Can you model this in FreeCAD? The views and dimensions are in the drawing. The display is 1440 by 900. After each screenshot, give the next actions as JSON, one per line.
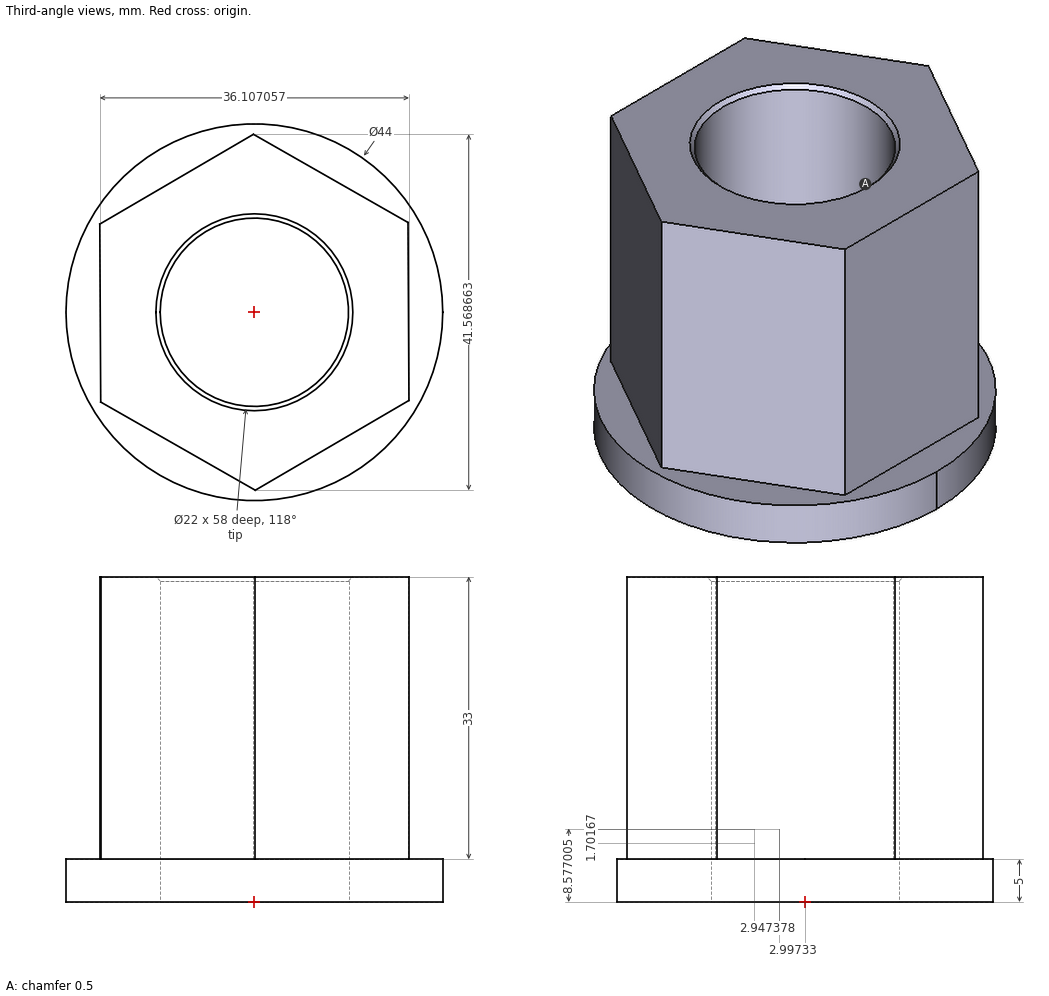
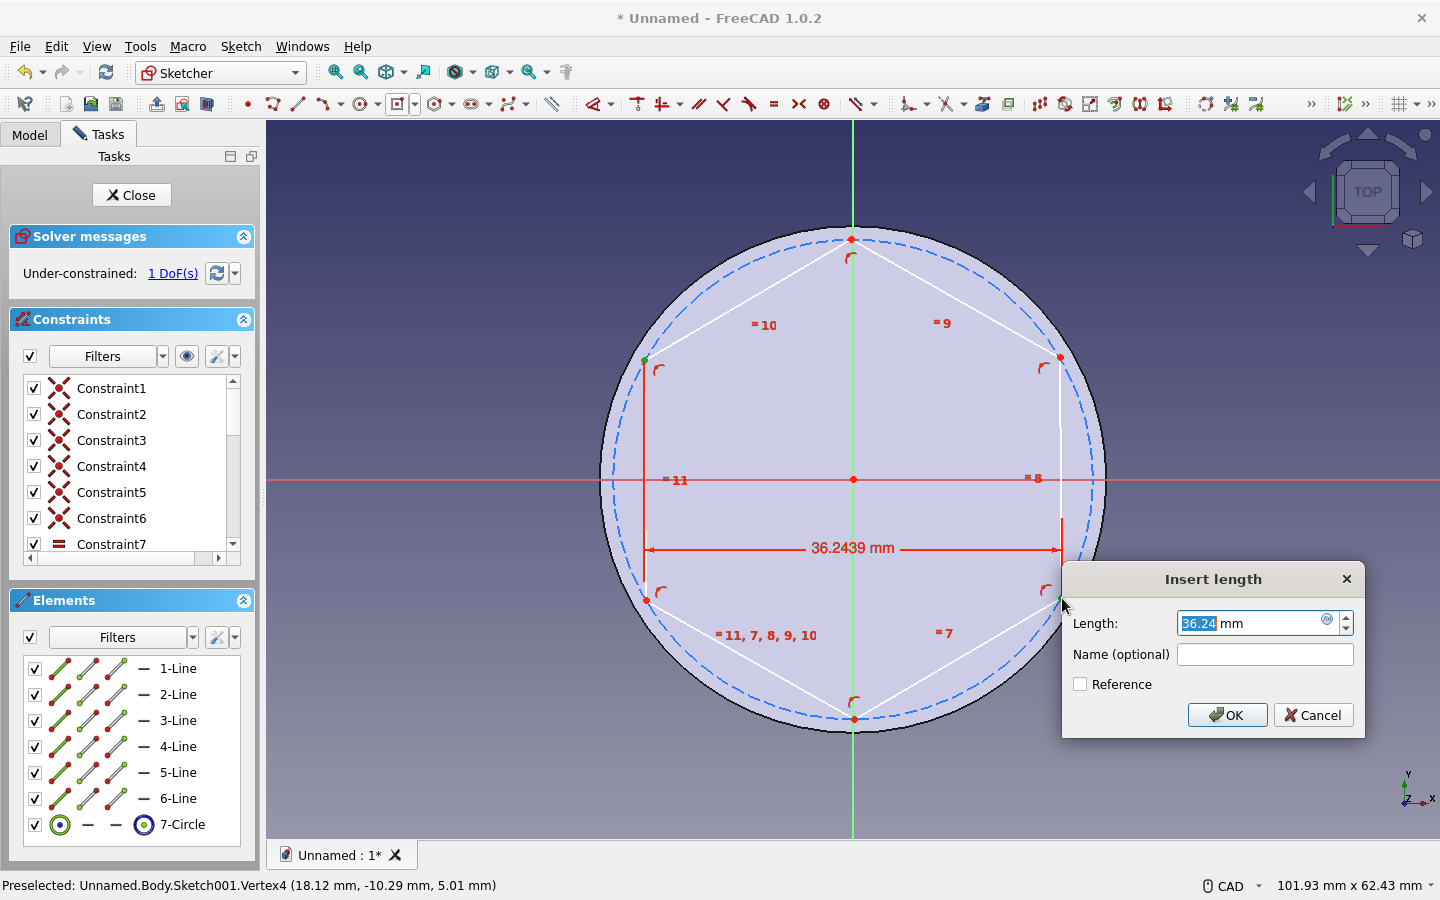
{"action": "type", "text": "36.107057"}
{"action": "key", "text": "Return"}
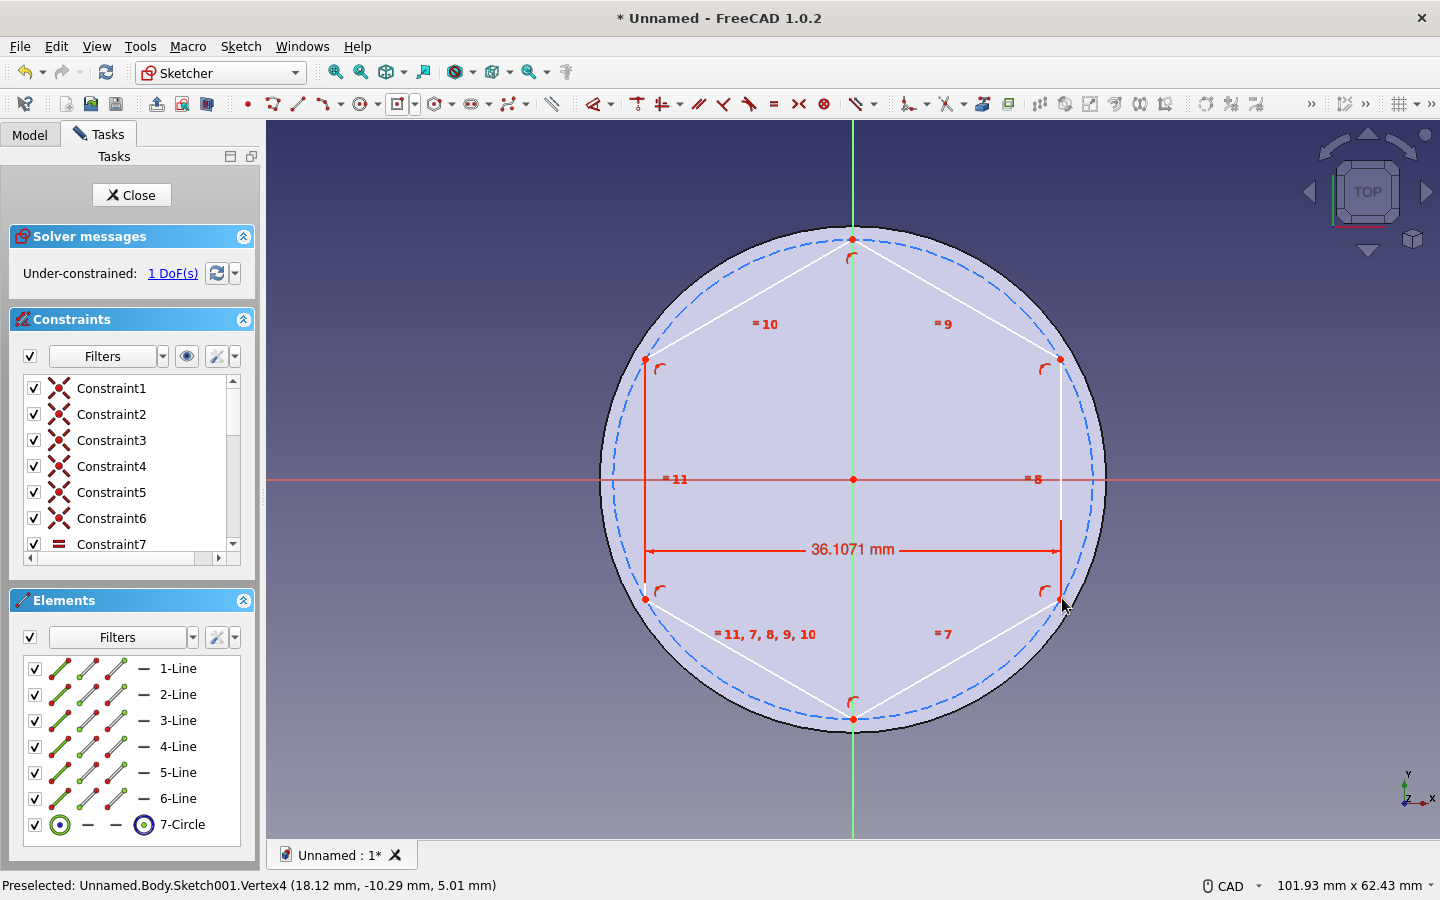
{"action": "left_click", "coordinate": [853, 720]}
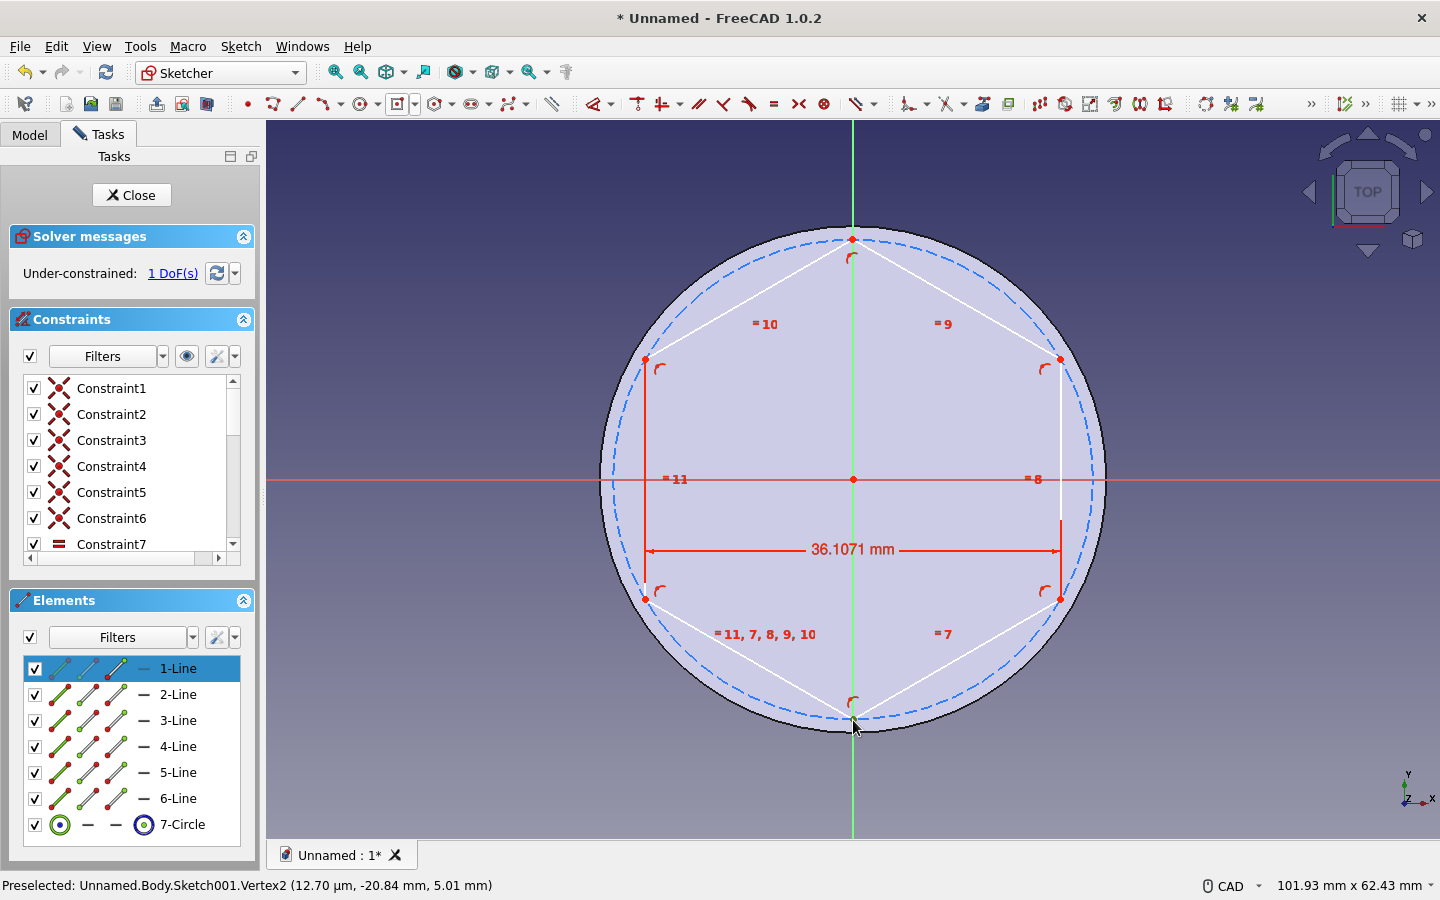
{"action": "left_click", "coordinate": [853, 239]}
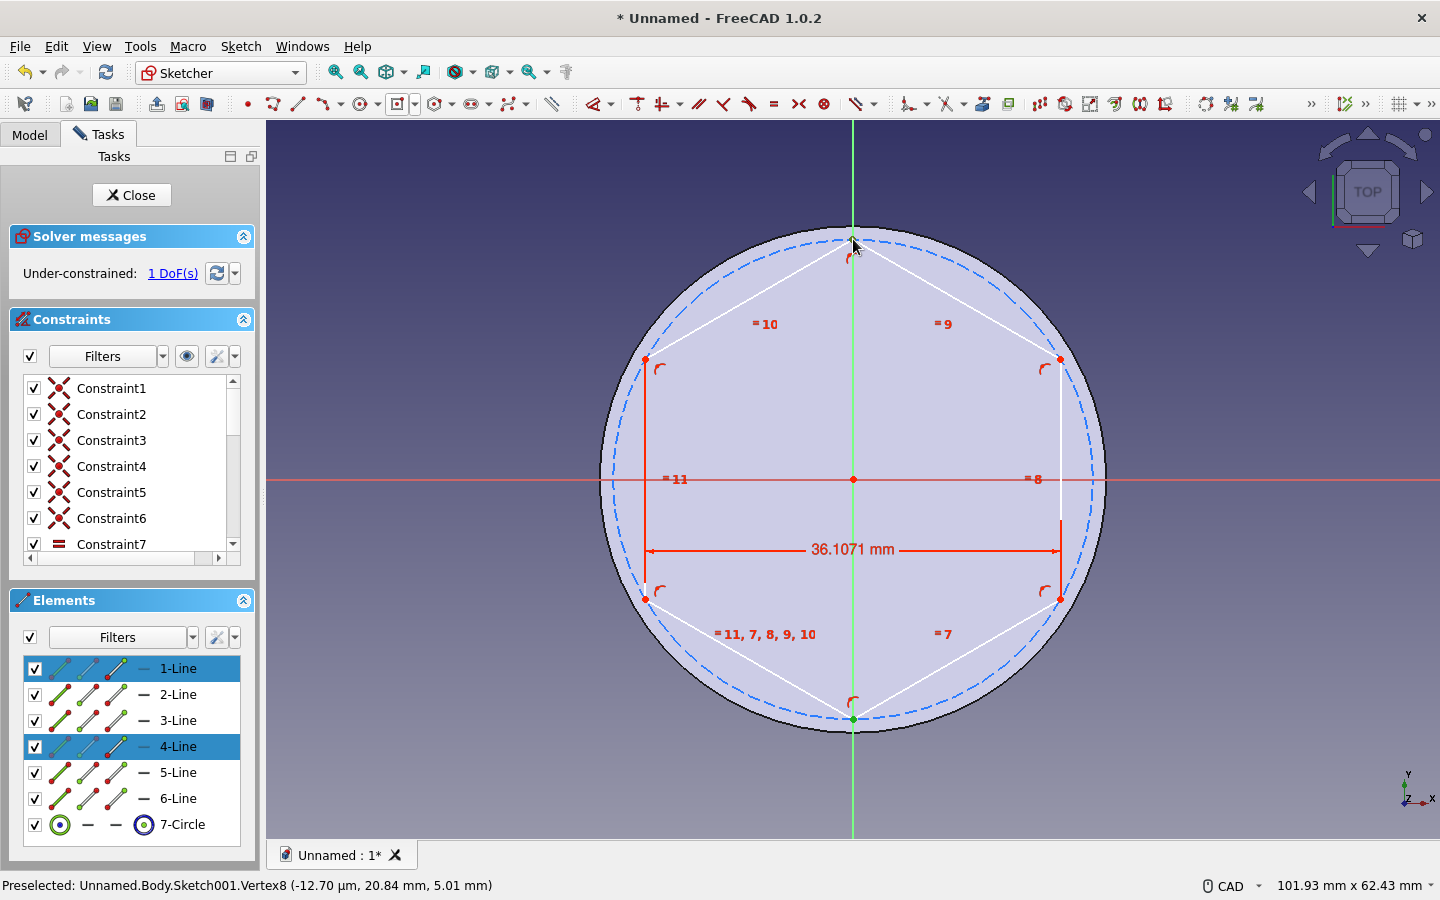
{"action": "key", "text": "i"}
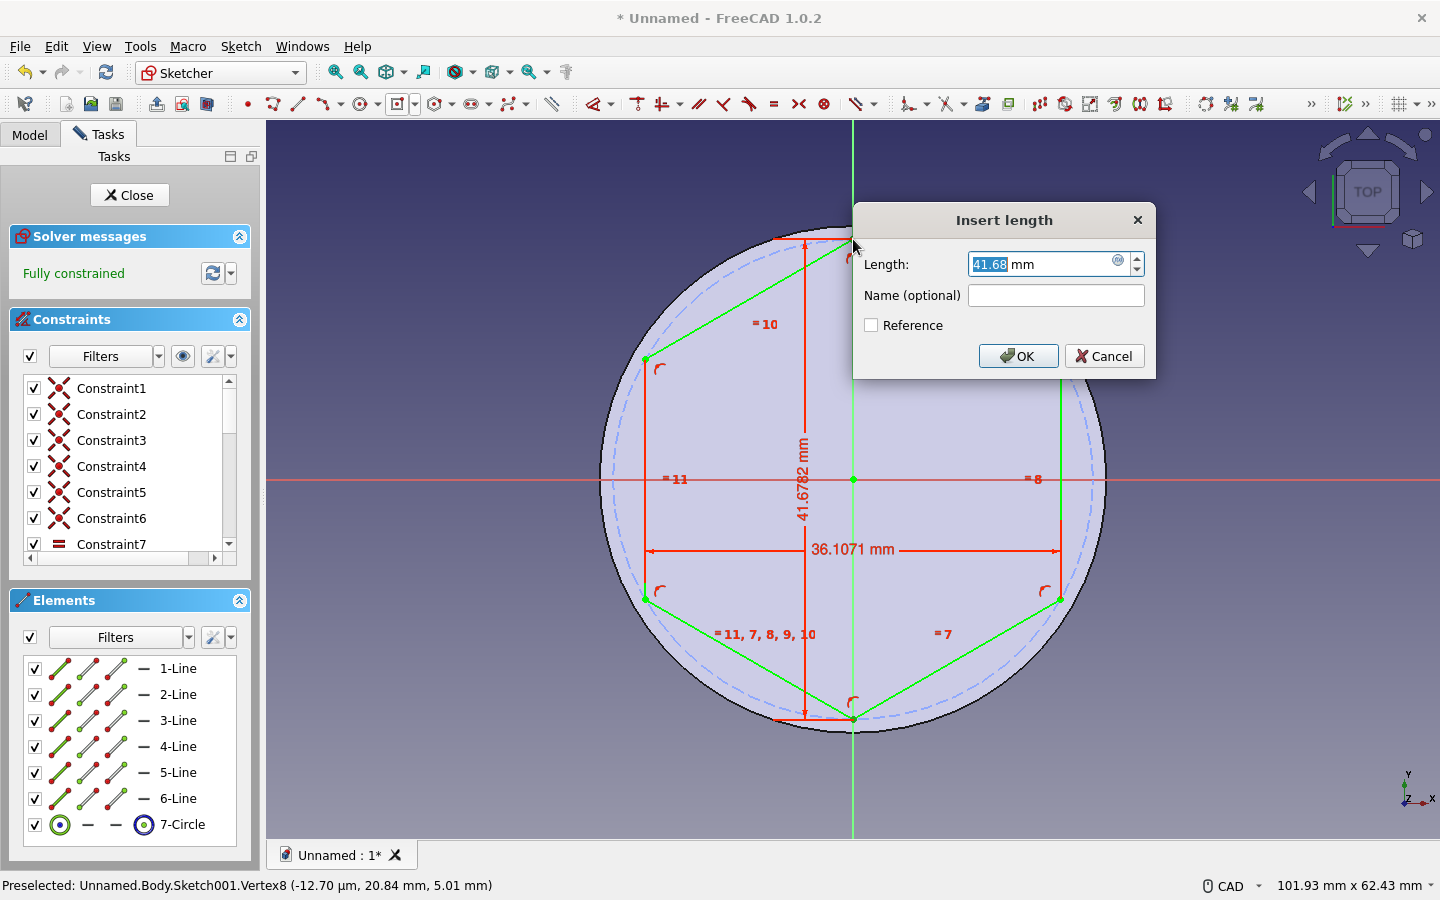
{"action": "type", "text": "41.568663"}
{"action": "key", "text": "Return"}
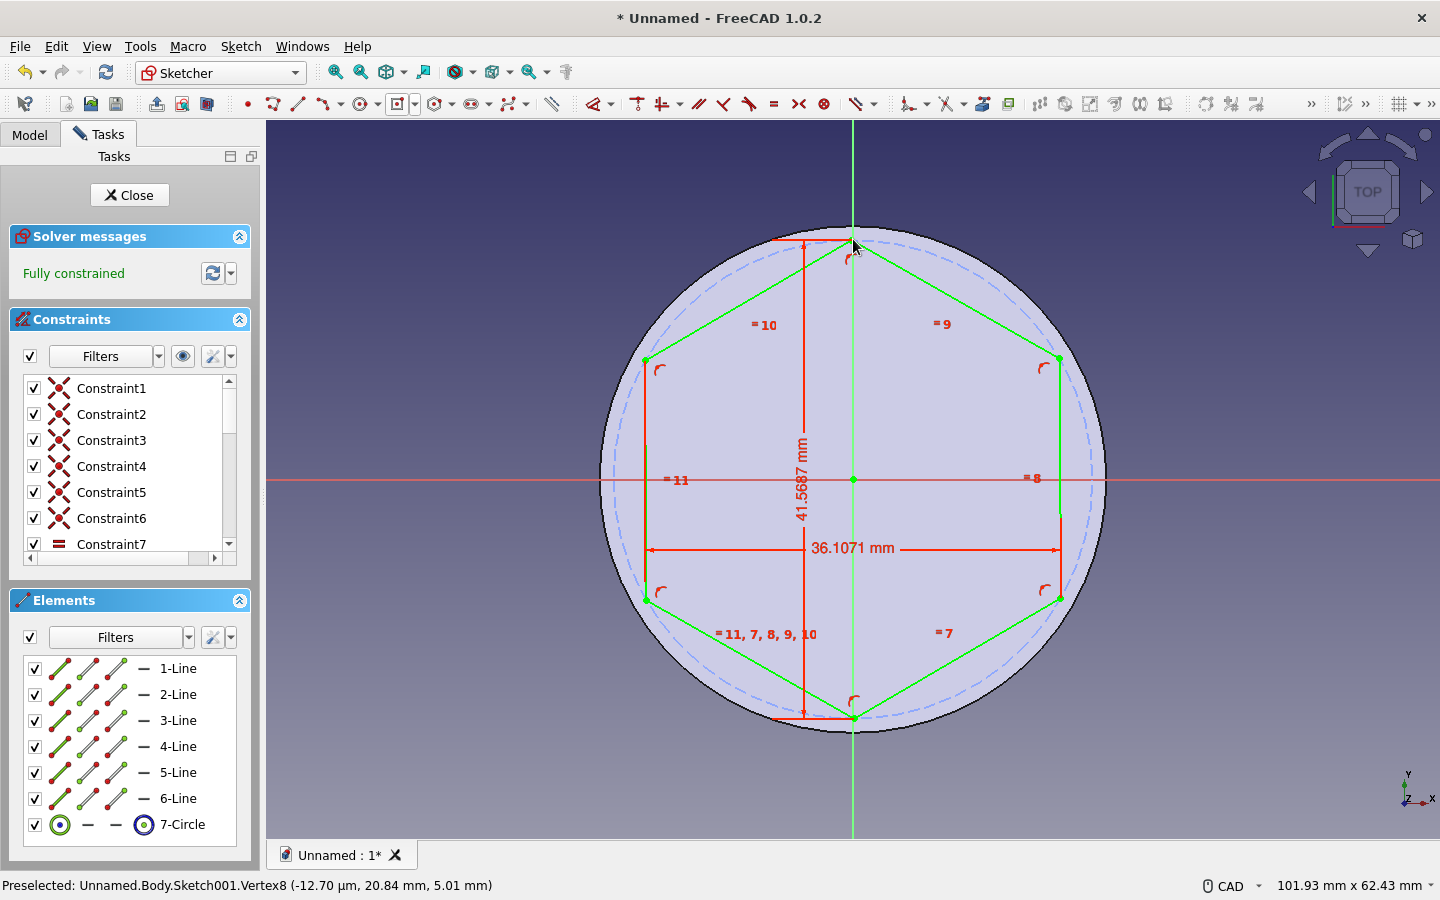
{"action": "left_click", "coordinate": [130, 195]}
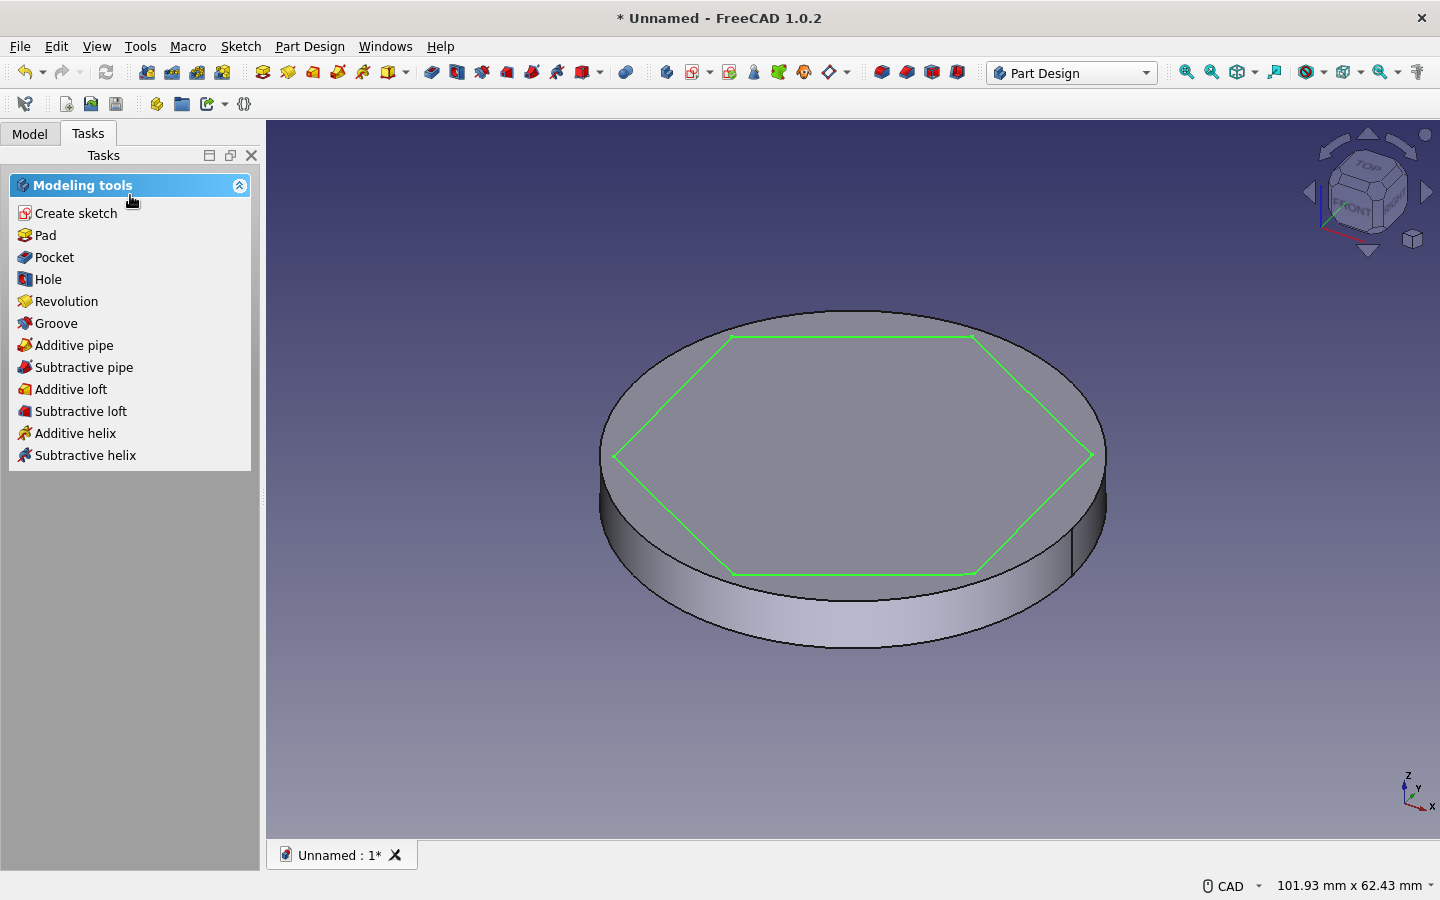
{"action": "left_click", "coordinate": [263, 72]}